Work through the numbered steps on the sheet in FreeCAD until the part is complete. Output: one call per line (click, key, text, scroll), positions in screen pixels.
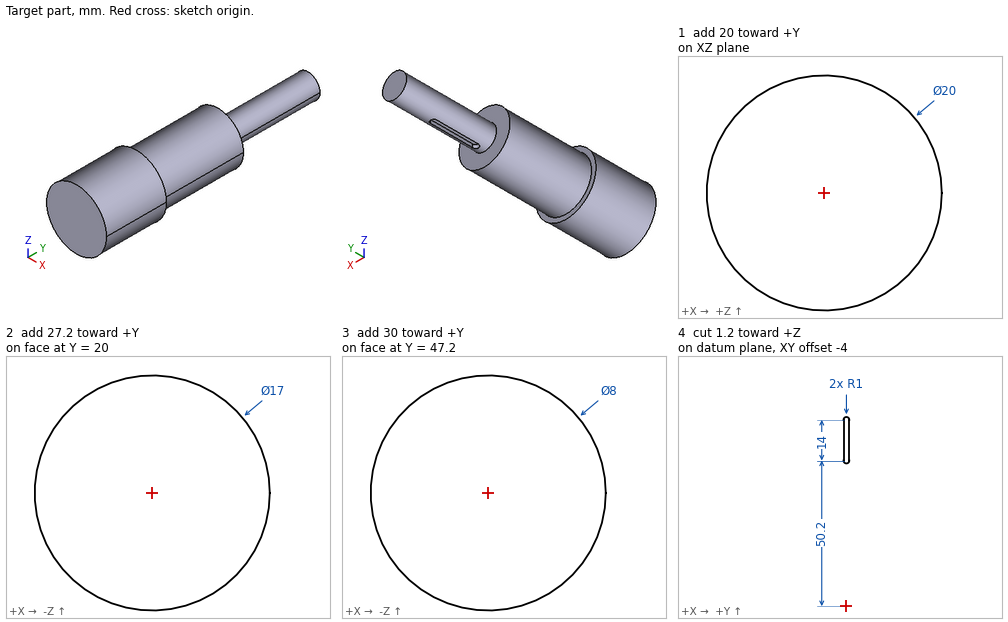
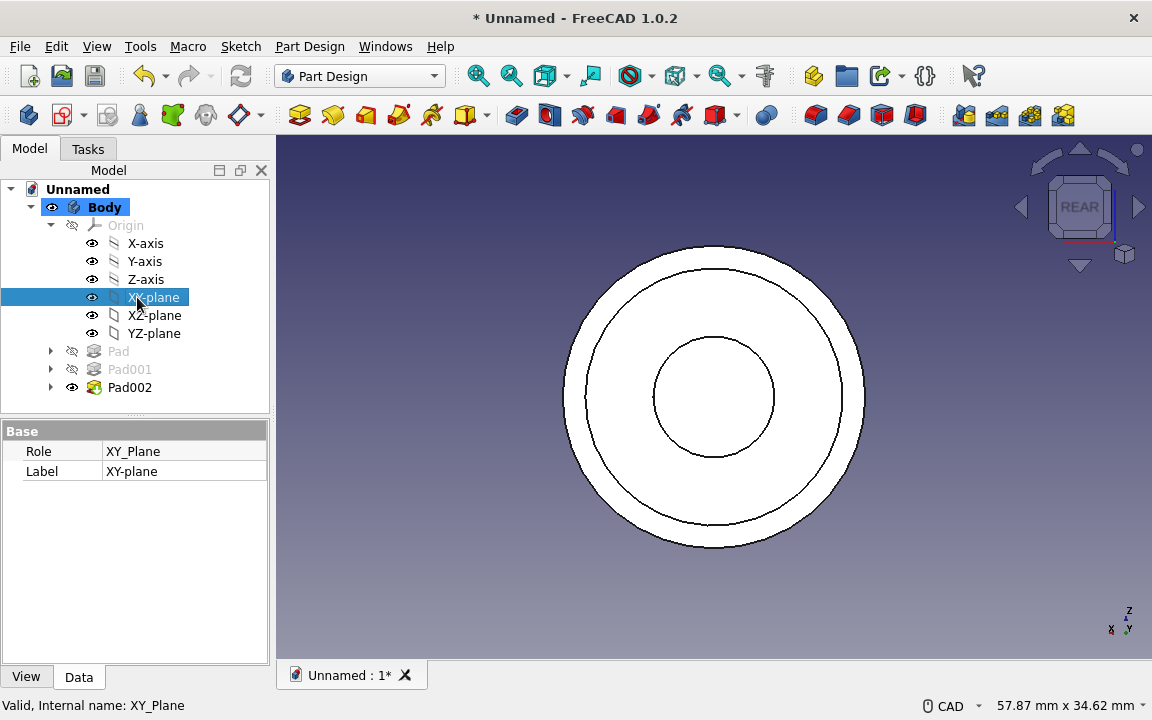
click(238, 116)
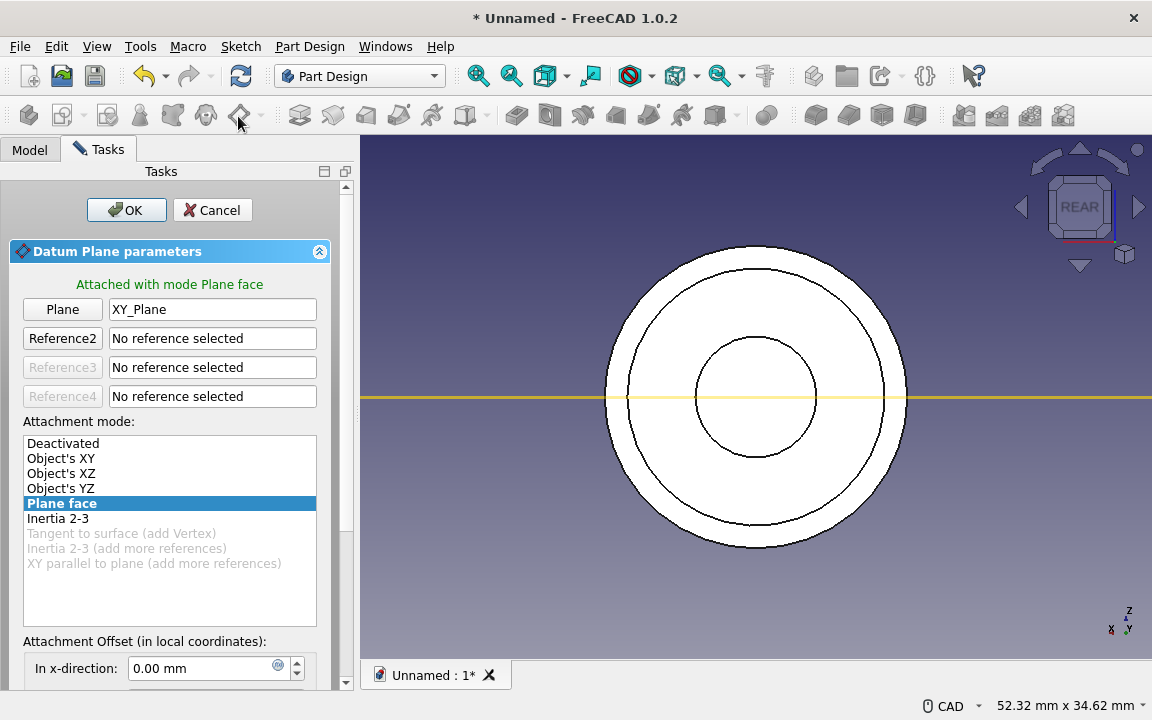
scroll(346, 436, down, 2)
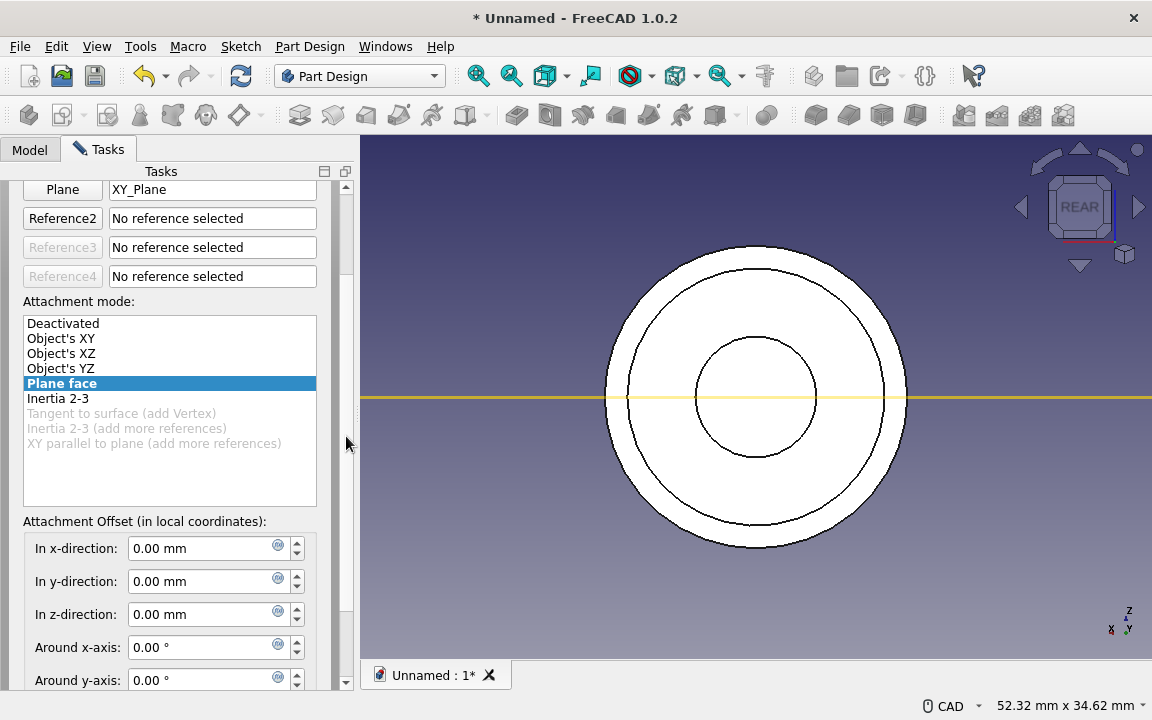
triple_click(210, 614)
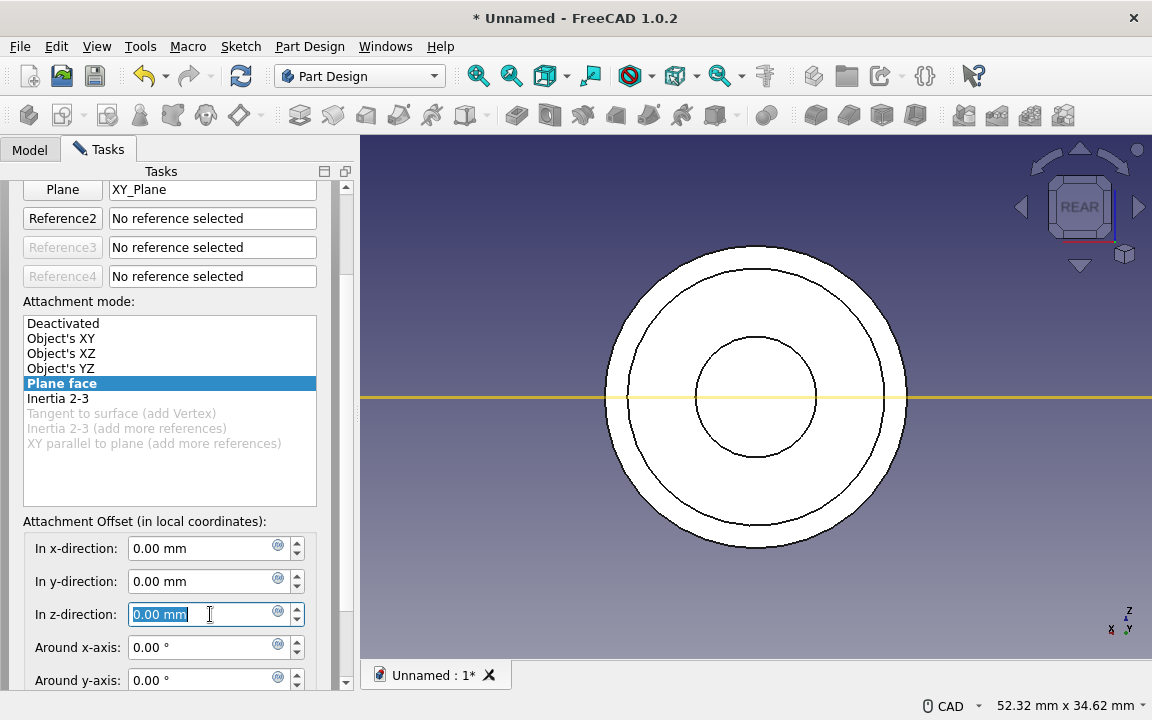
text(-4)
key(Tab)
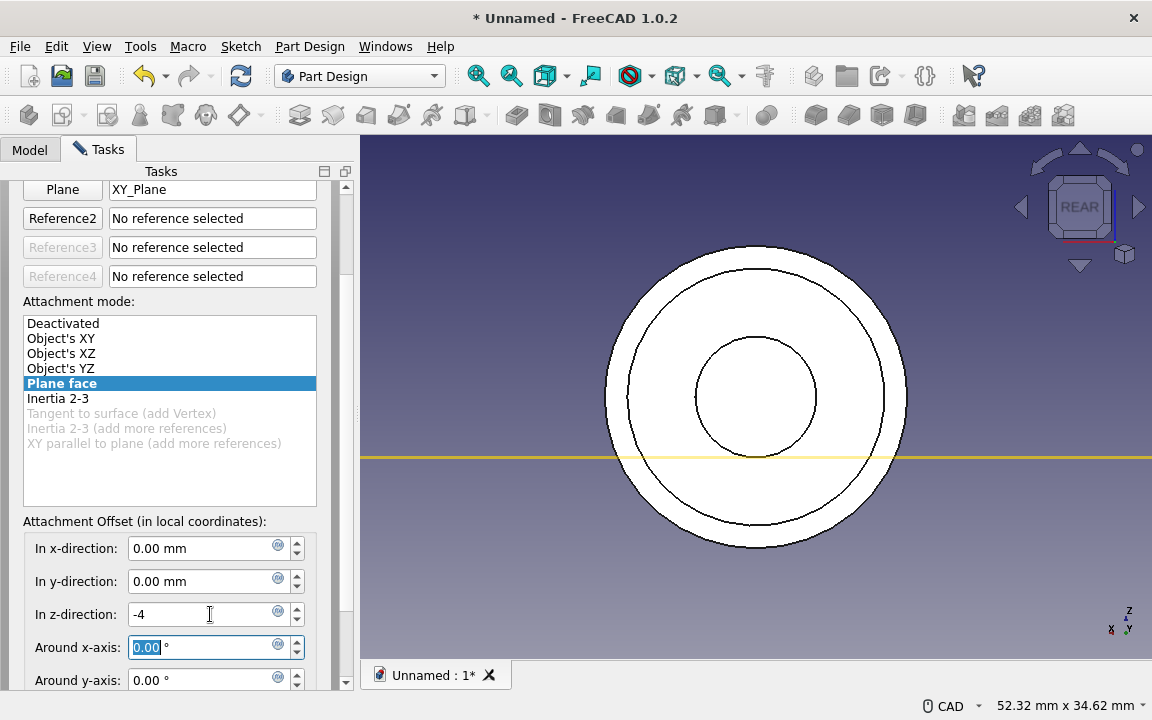
scroll(346, 436, up, 3)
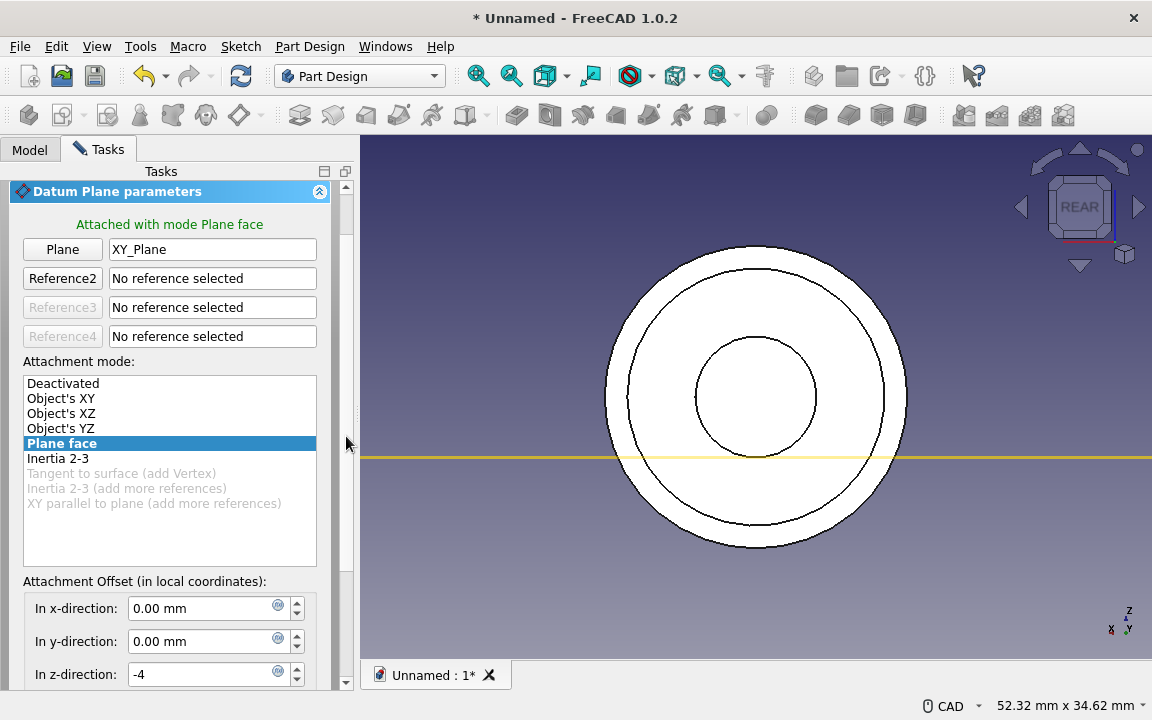
click(127, 210)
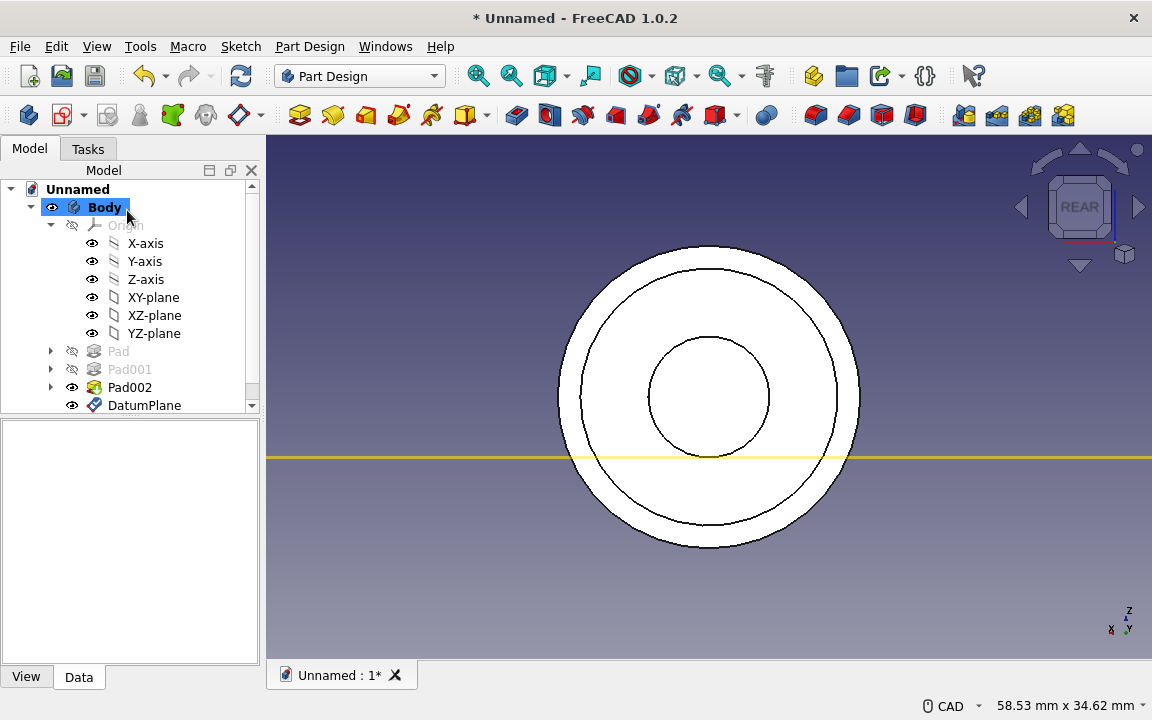
click(117, 405)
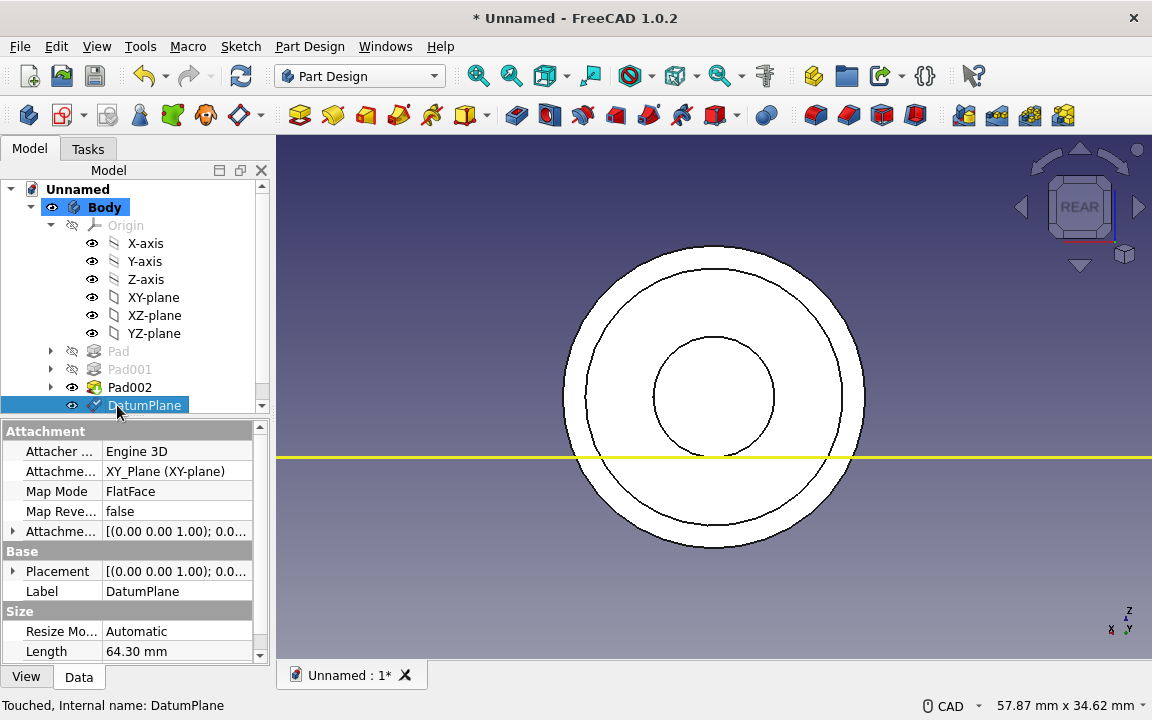
click(62, 116)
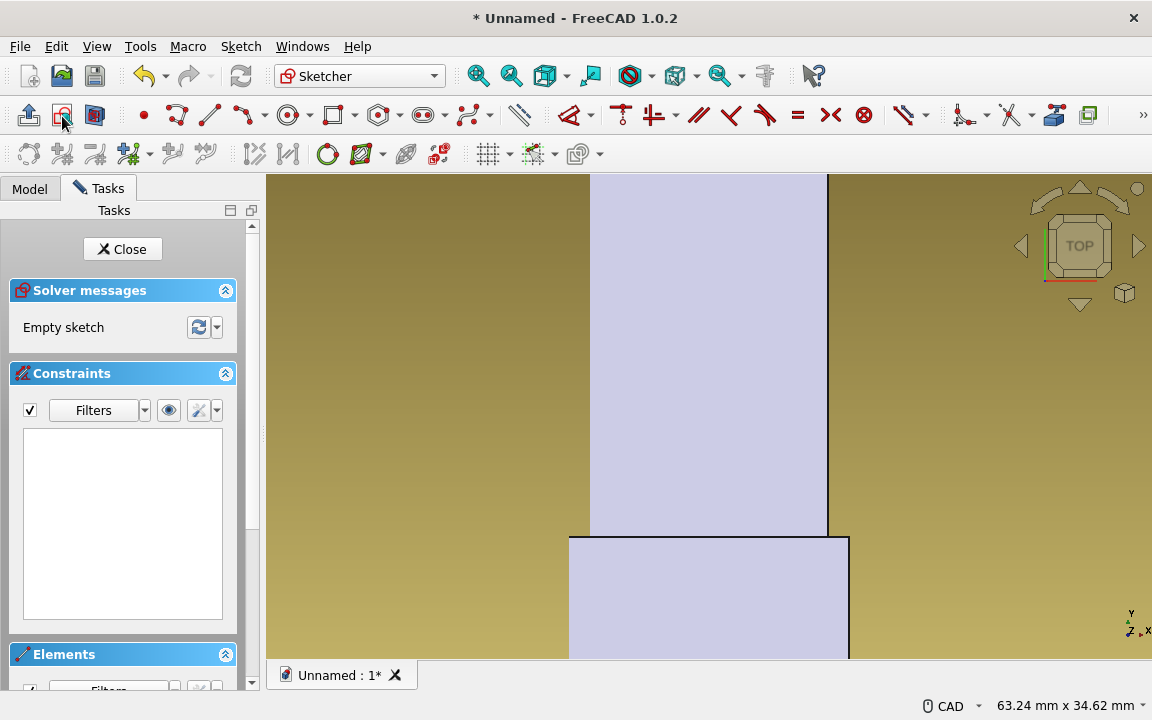
click(95, 116)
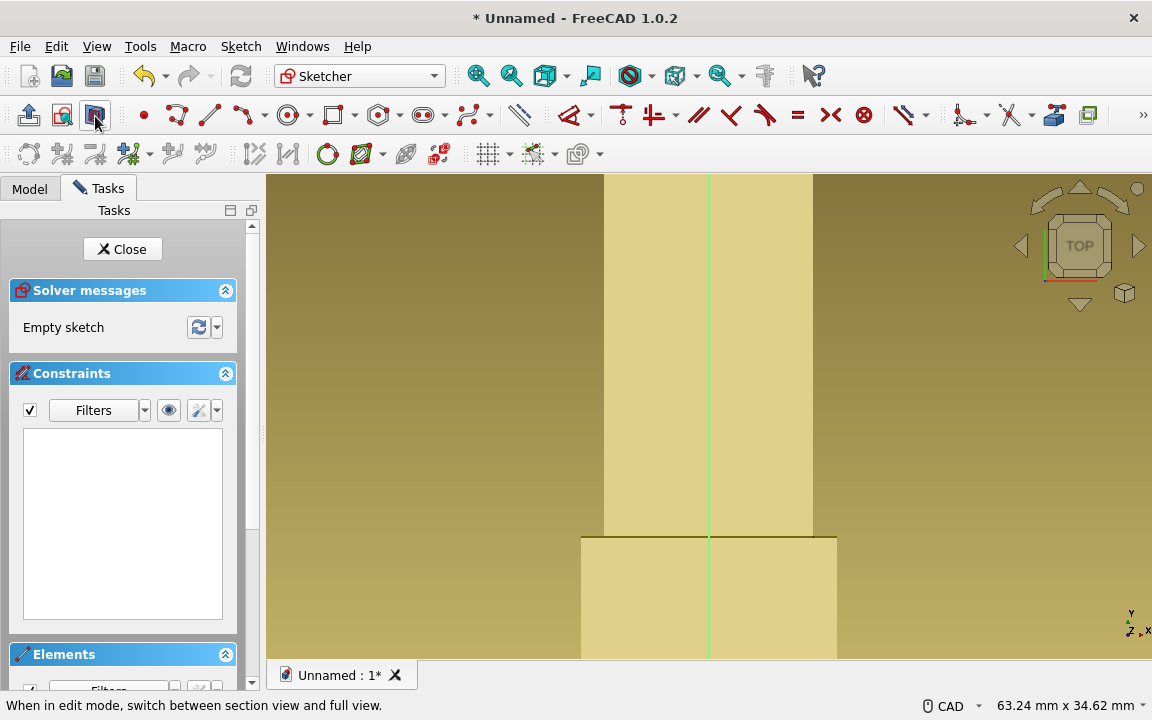
scroll(640, 416, down, 5)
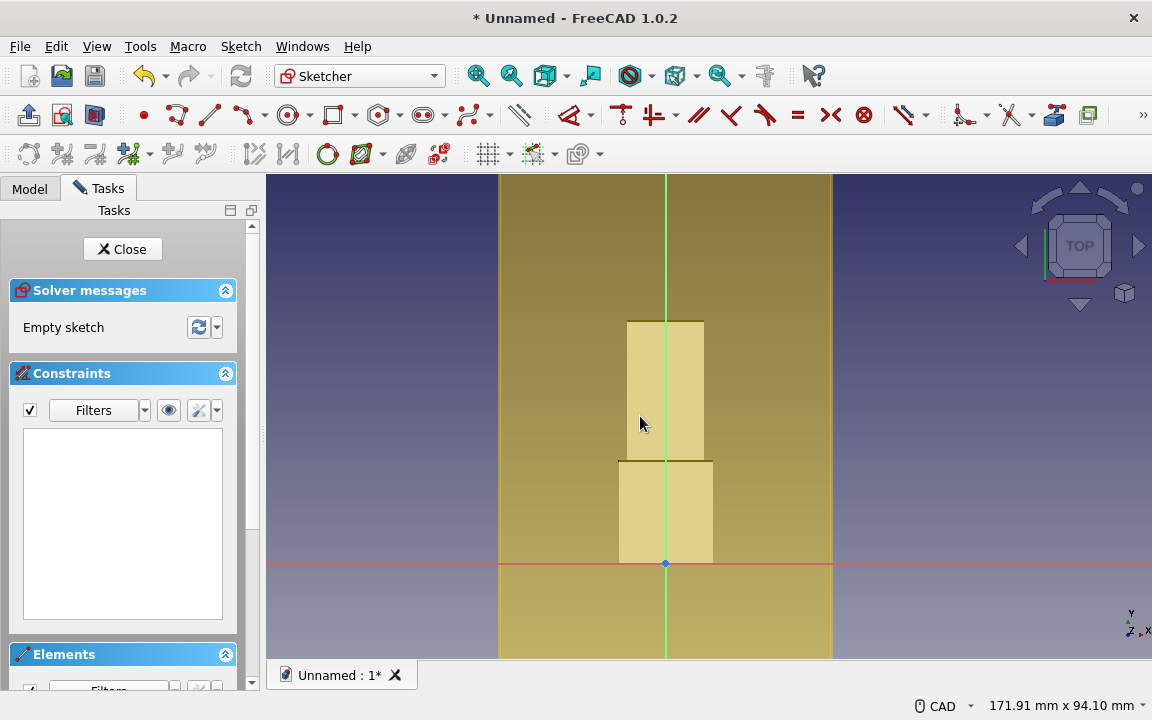
scroll(674, 221, up, 7)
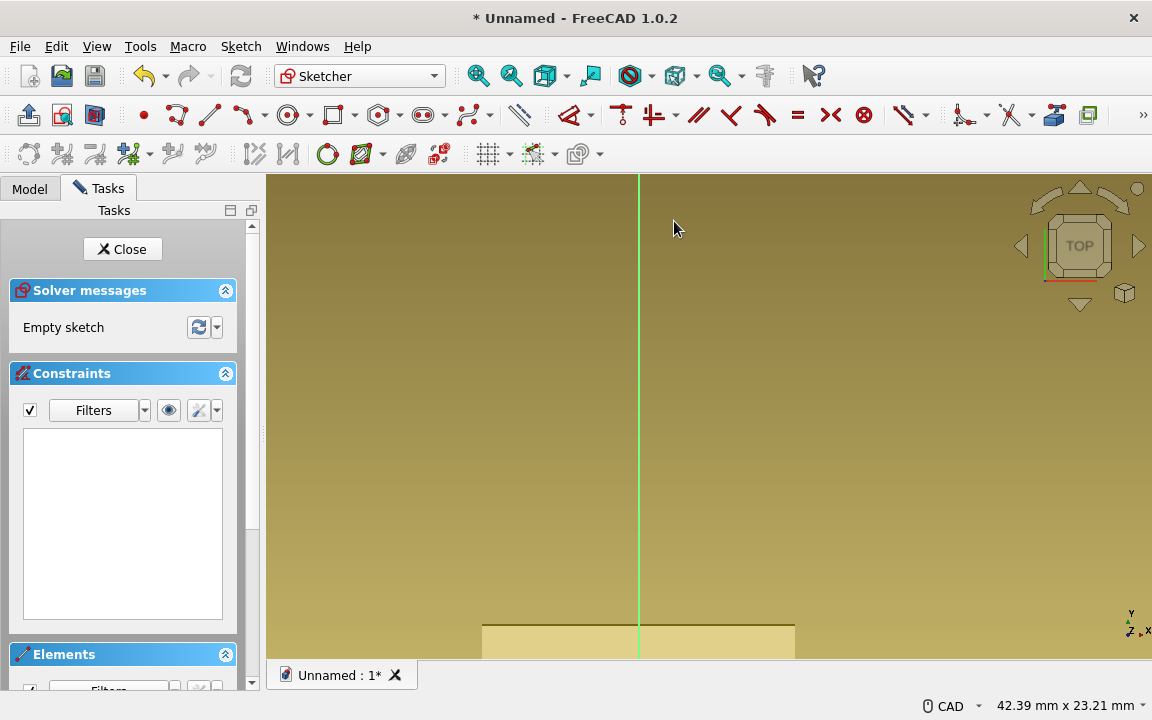
key(g)
key(s)